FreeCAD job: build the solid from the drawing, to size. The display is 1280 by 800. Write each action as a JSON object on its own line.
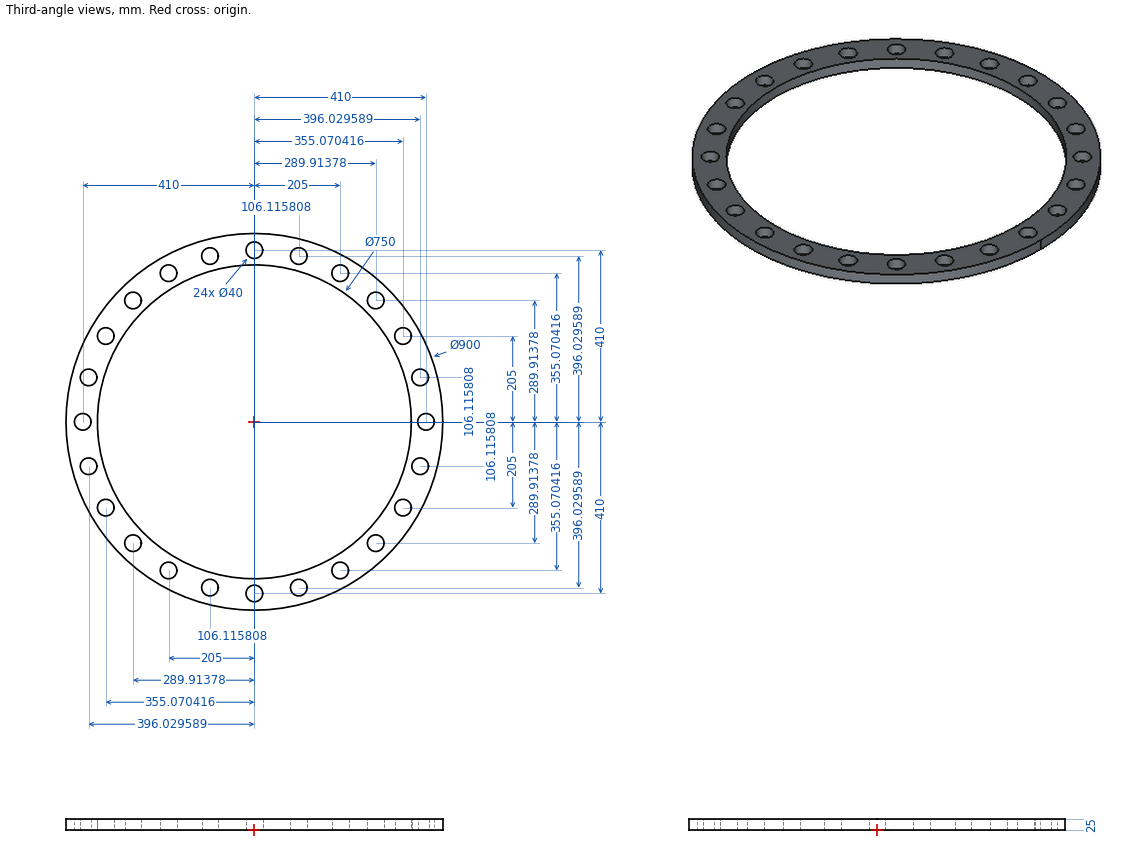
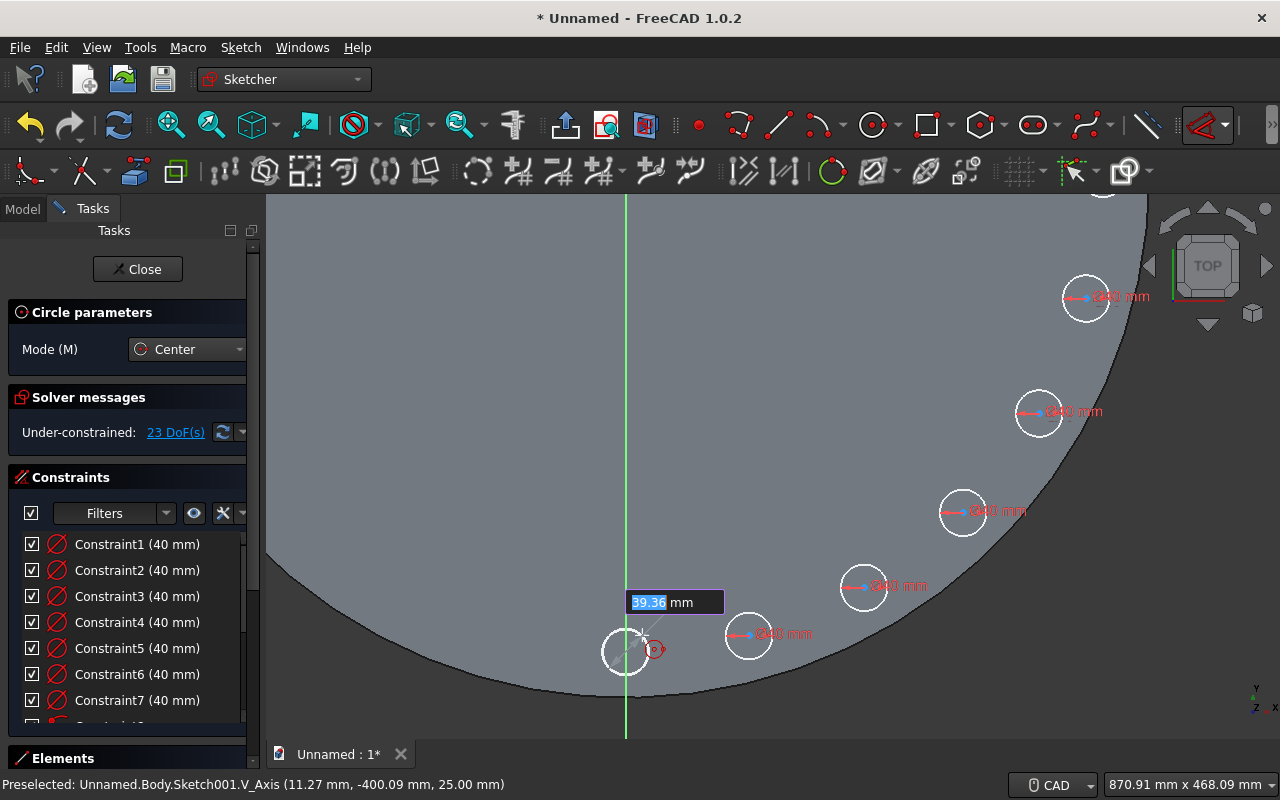
{"action": "type", "text": "40"}
{"action": "key", "text": "Return"}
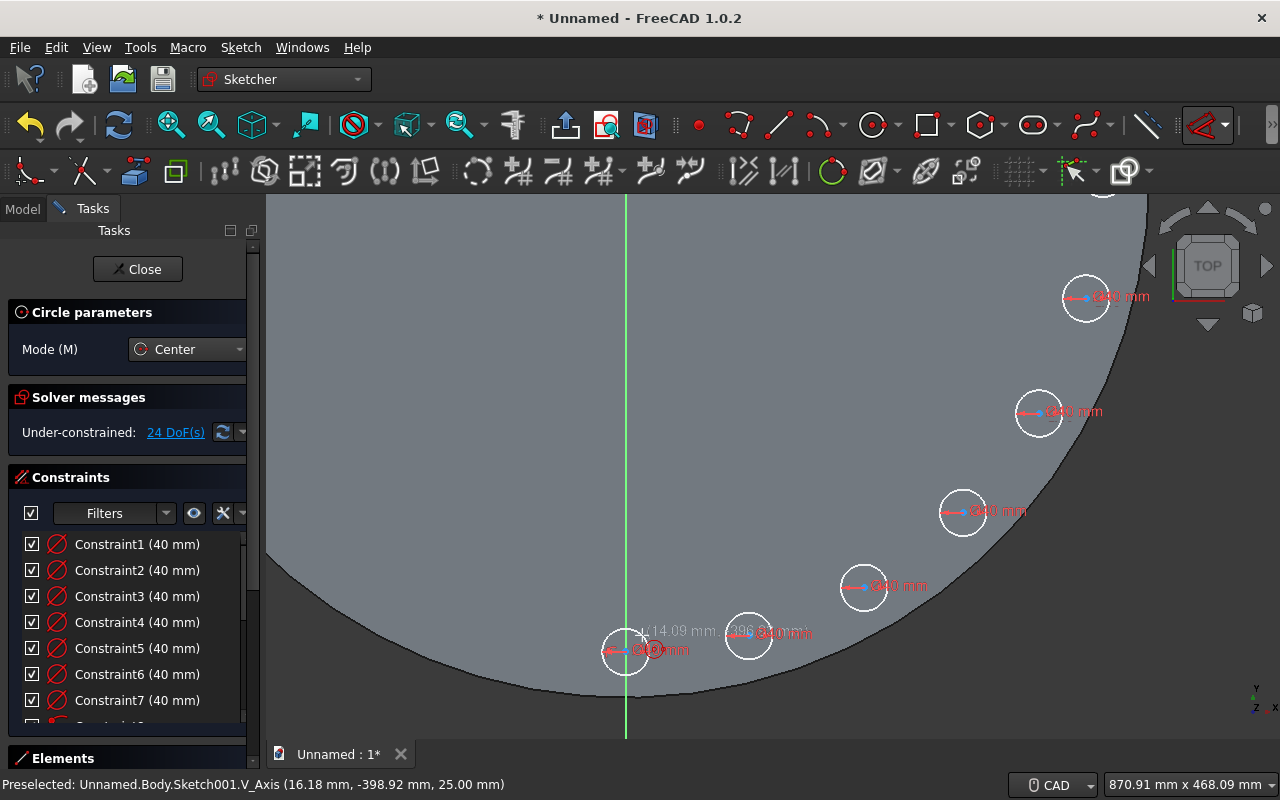
{"action": "left_click", "coordinate": [502, 635]}
{"action": "mouse_move", "coordinate": [519, 618]}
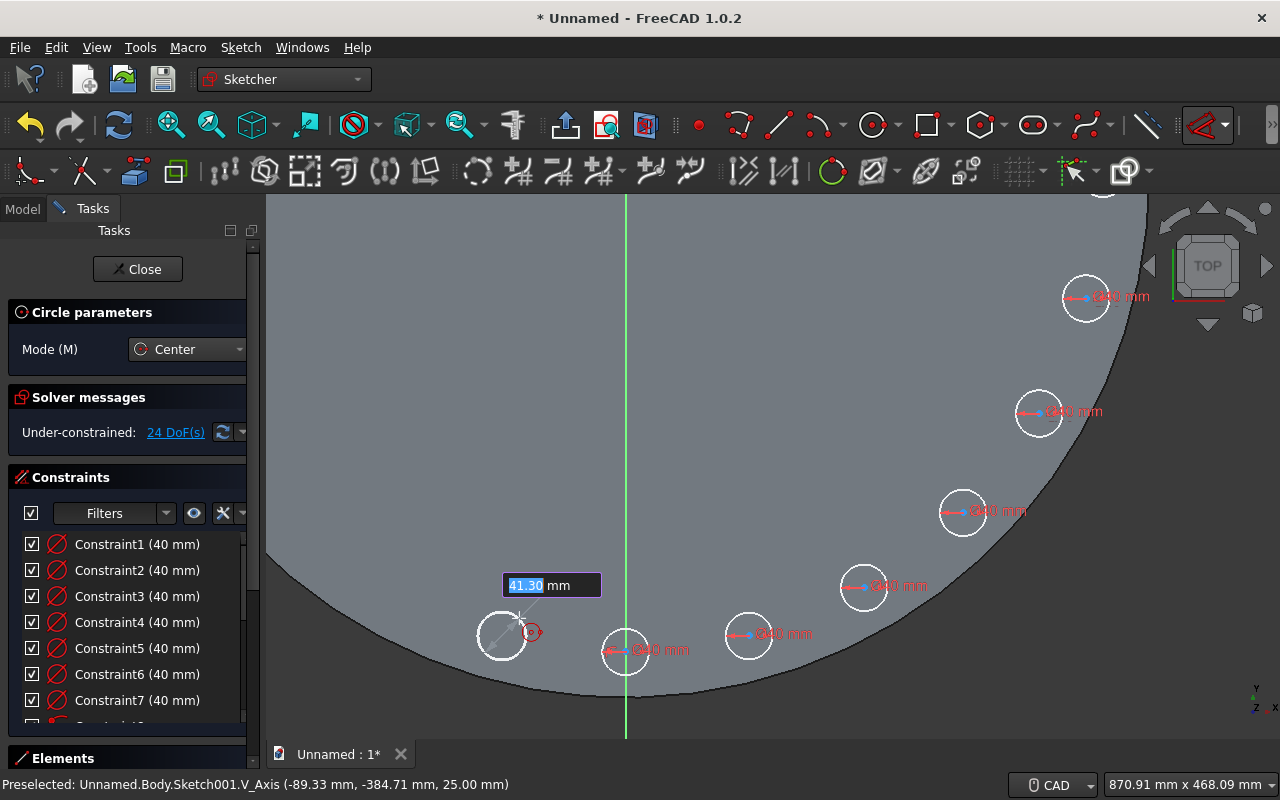
{"action": "type", "text": "40"}
{"action": "key", "text": "Return"}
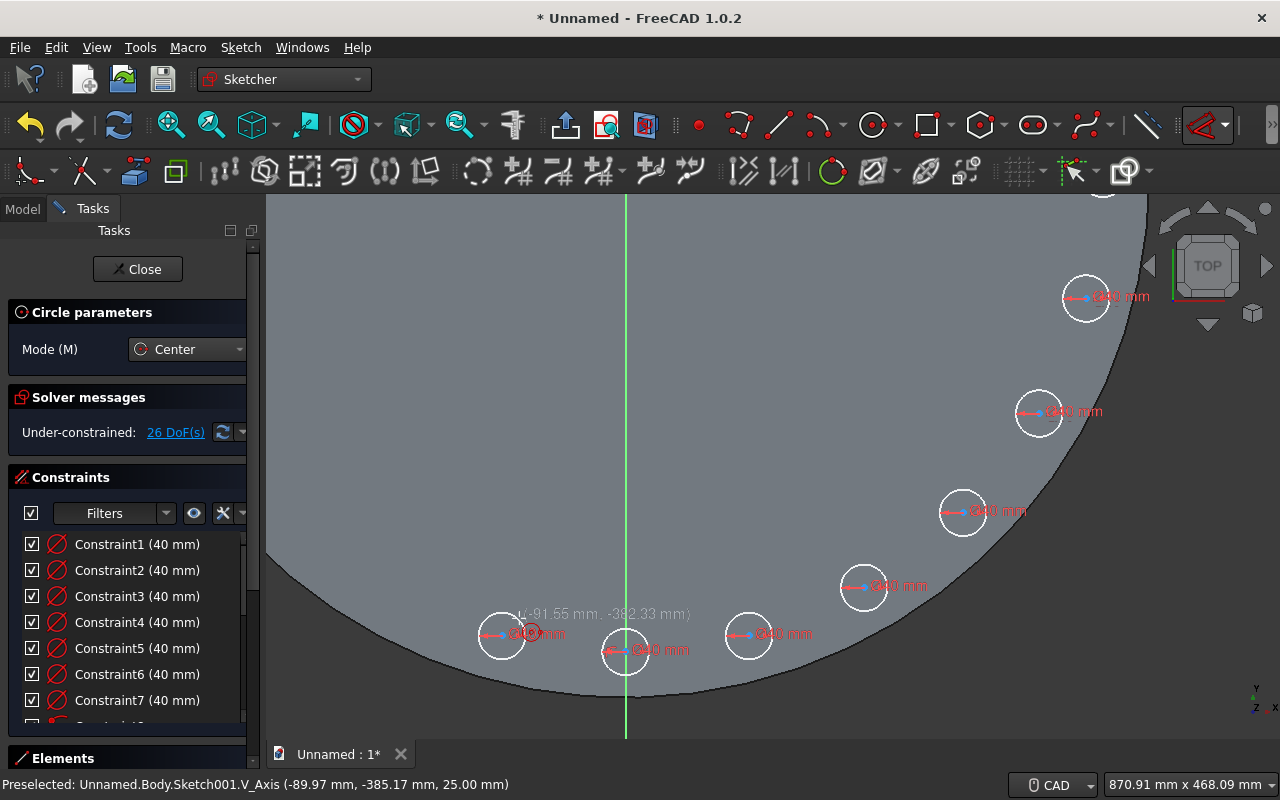
{"action": "left_click", "coordinate": [387, 587]}
{"action": "mouse_move", "coordinate": [403, 571]}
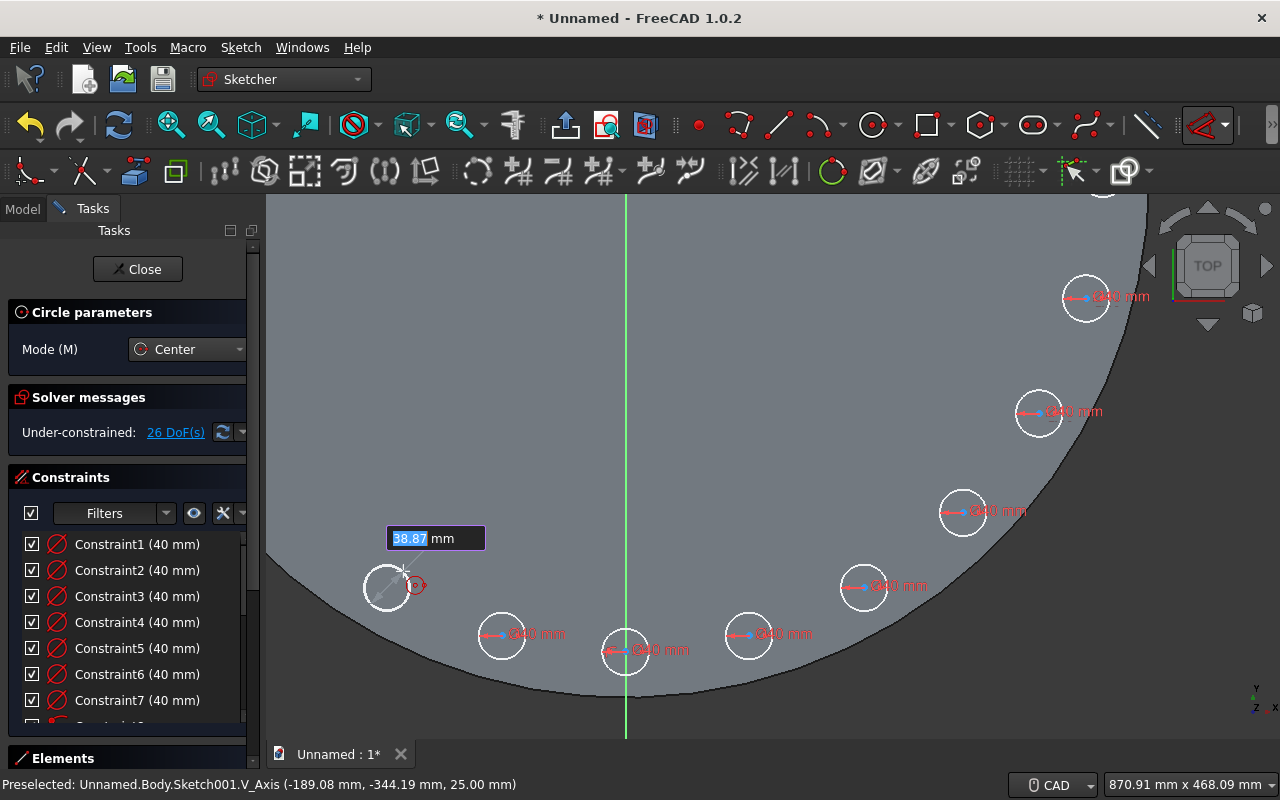
{"action": "type", "text": "40"}
{"action": "key", "text": "Return"}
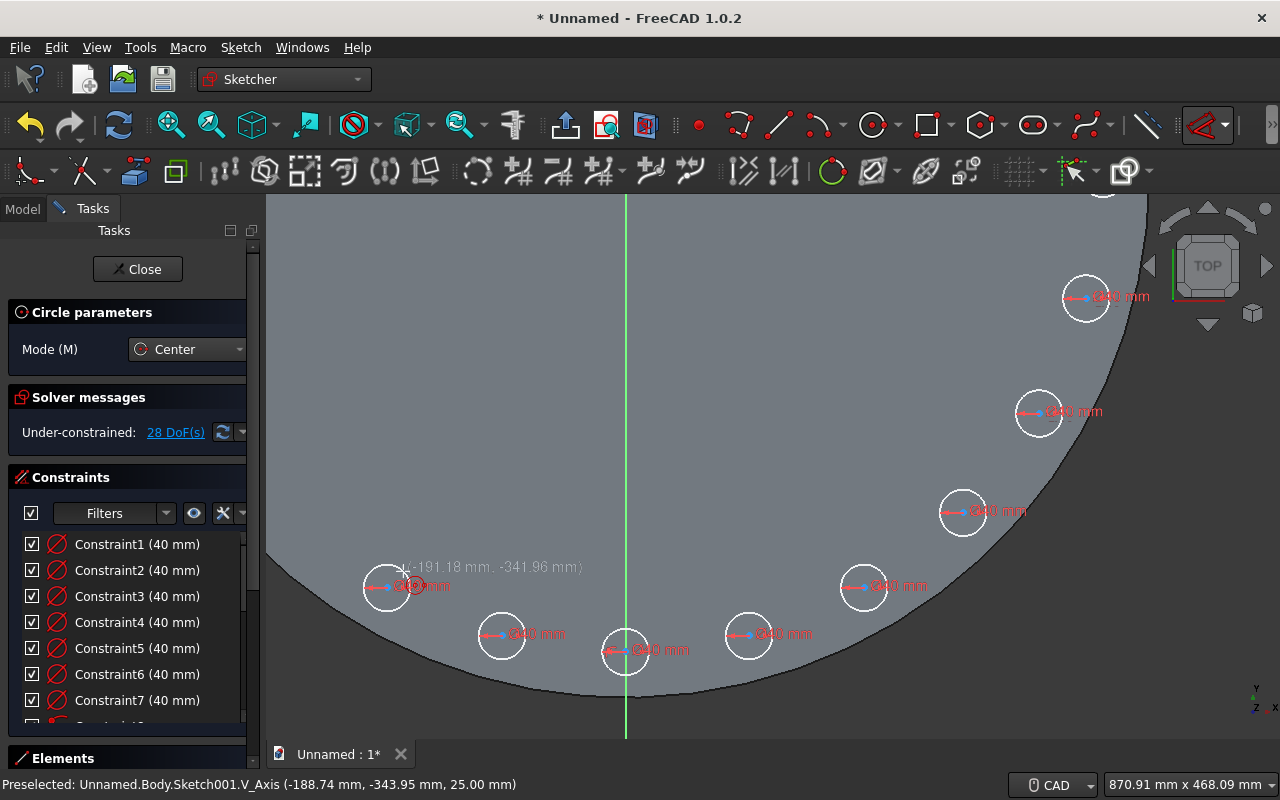
{"action": "scroll", "coordinate": [750, 637], "scroll_direction": "down", "scroll_amount": 5}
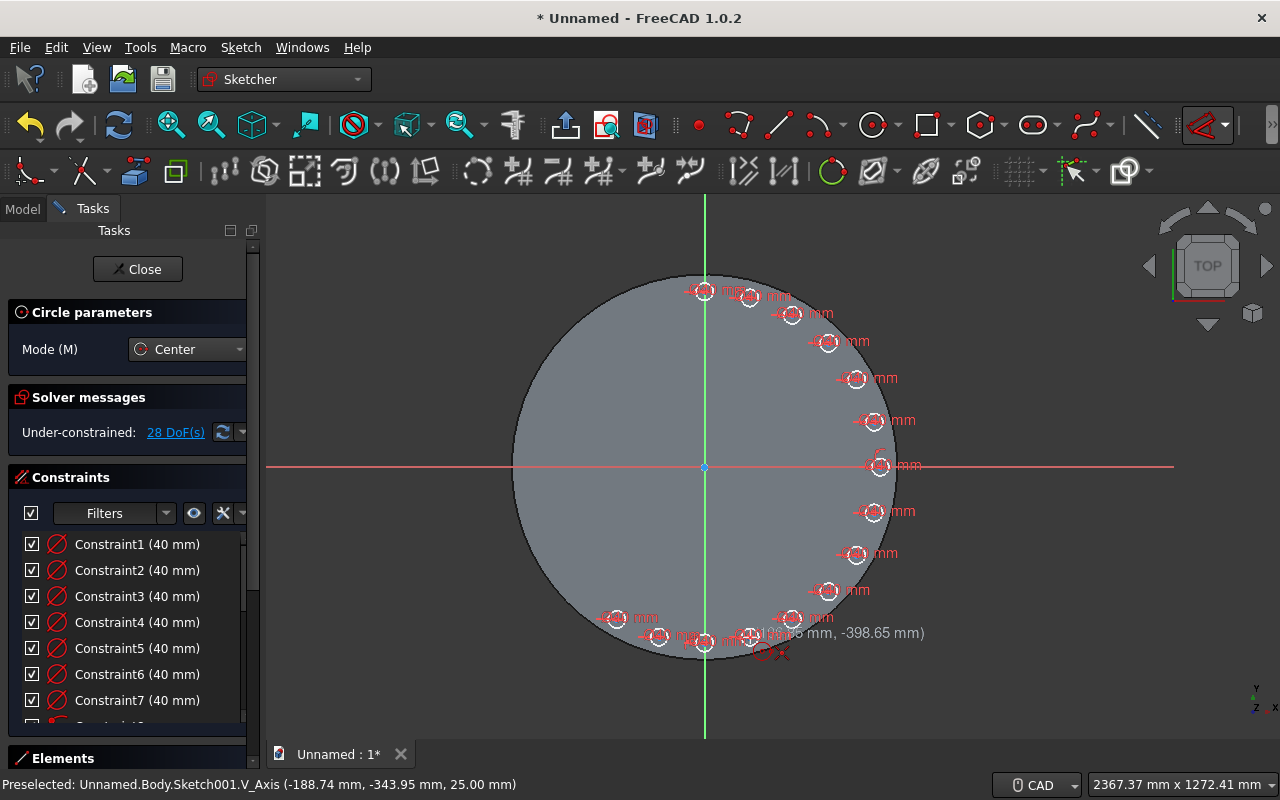
{"action": "scroll", "coordinate": [580, 591], "scroll_direction": "up", "scroll_amount": 5}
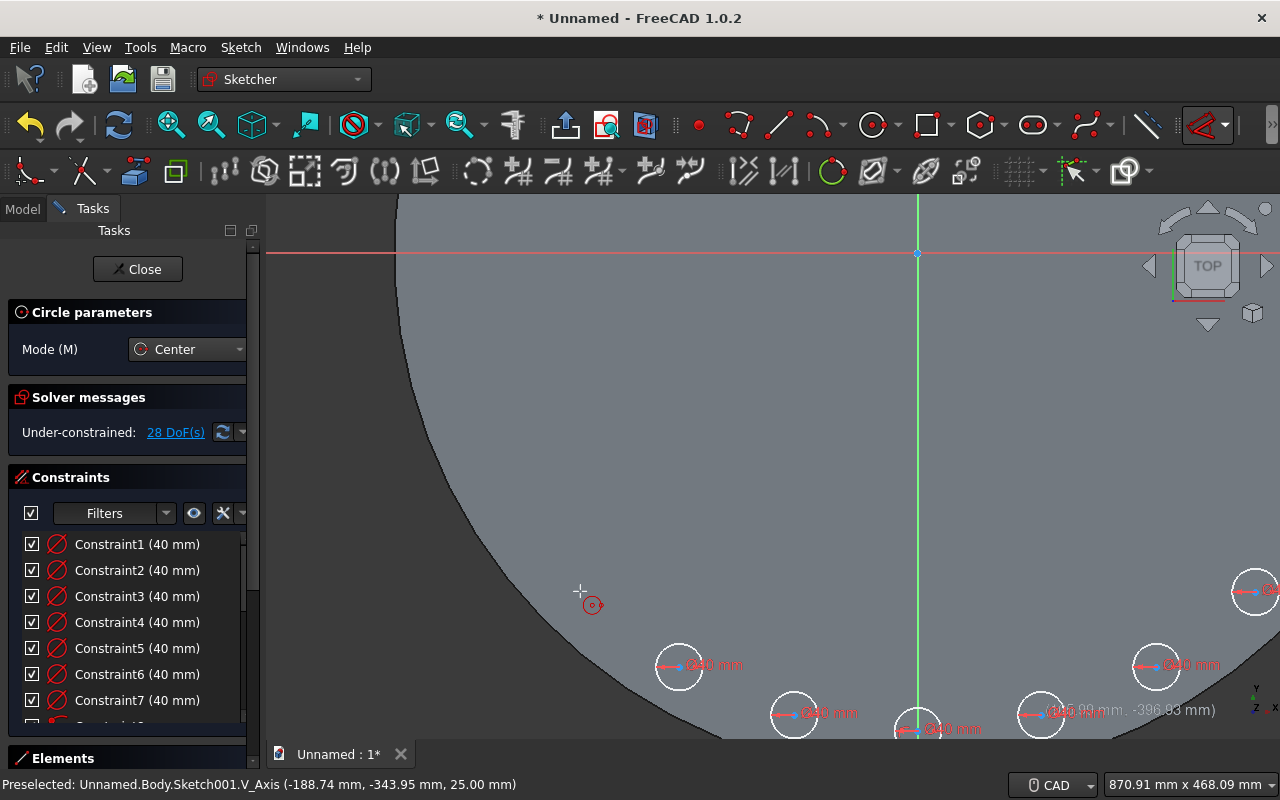
{"action": "left_click", "coordinate": [580, 591]}
{"action": "mouse_move", "coordinate": [597, 574]}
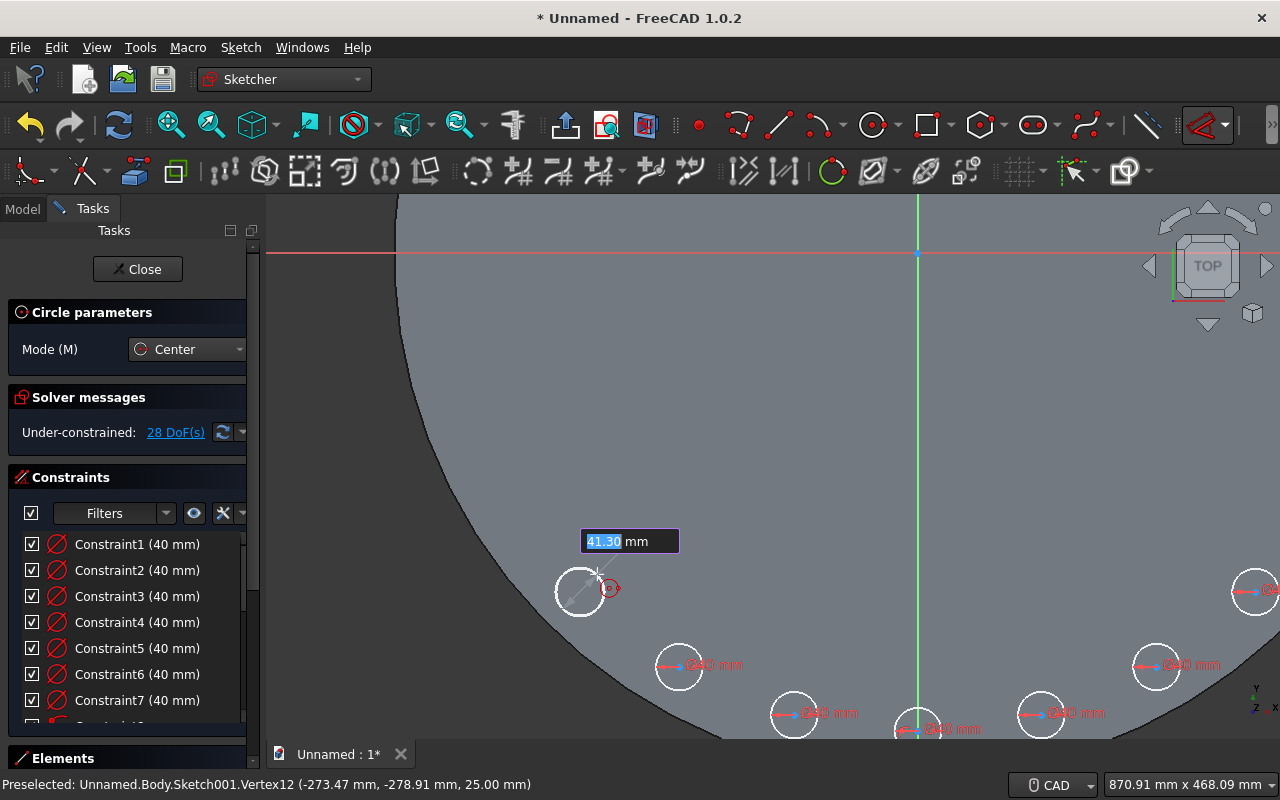
{"action": "type", "text": "40"}
{"action": "key", "text": "Return"}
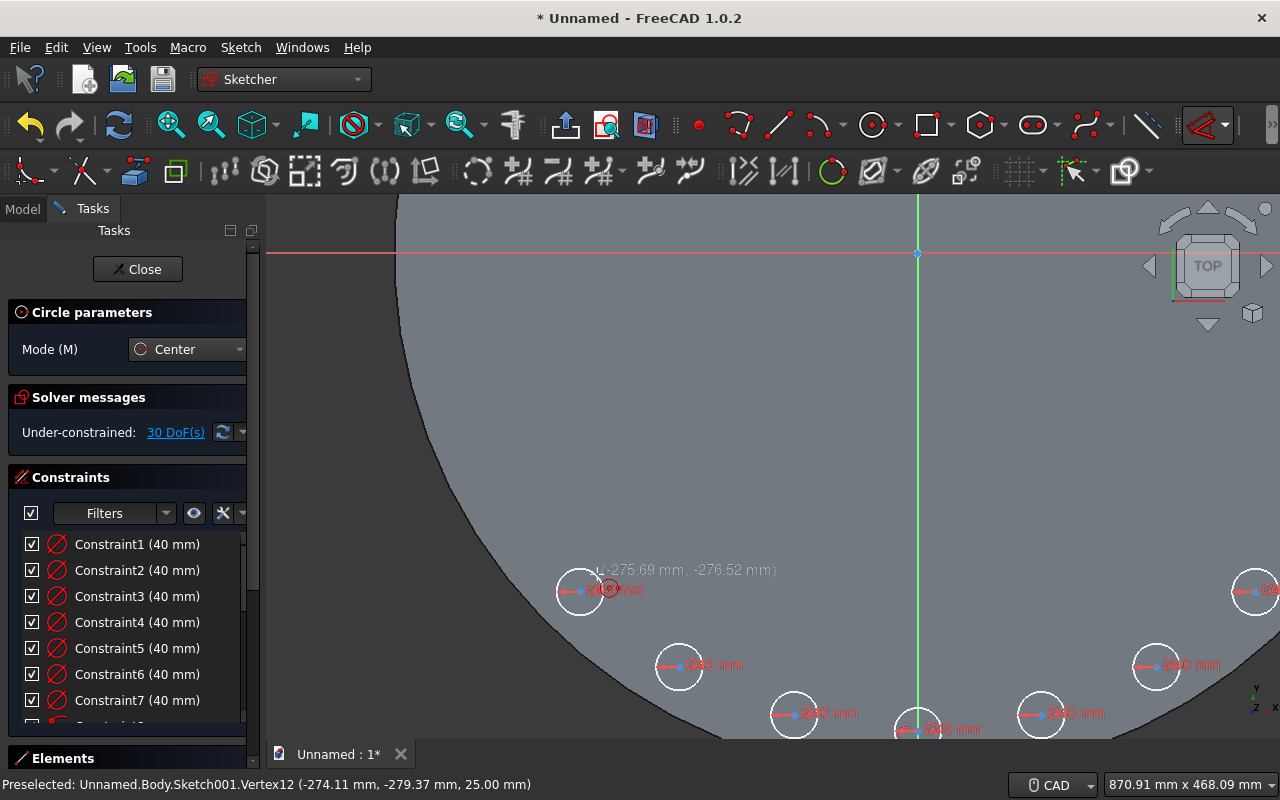
{"action": "left_click", "coordinate": [505, 492]}
{"action": "mouse_move", "coordinate": [521, 475]}